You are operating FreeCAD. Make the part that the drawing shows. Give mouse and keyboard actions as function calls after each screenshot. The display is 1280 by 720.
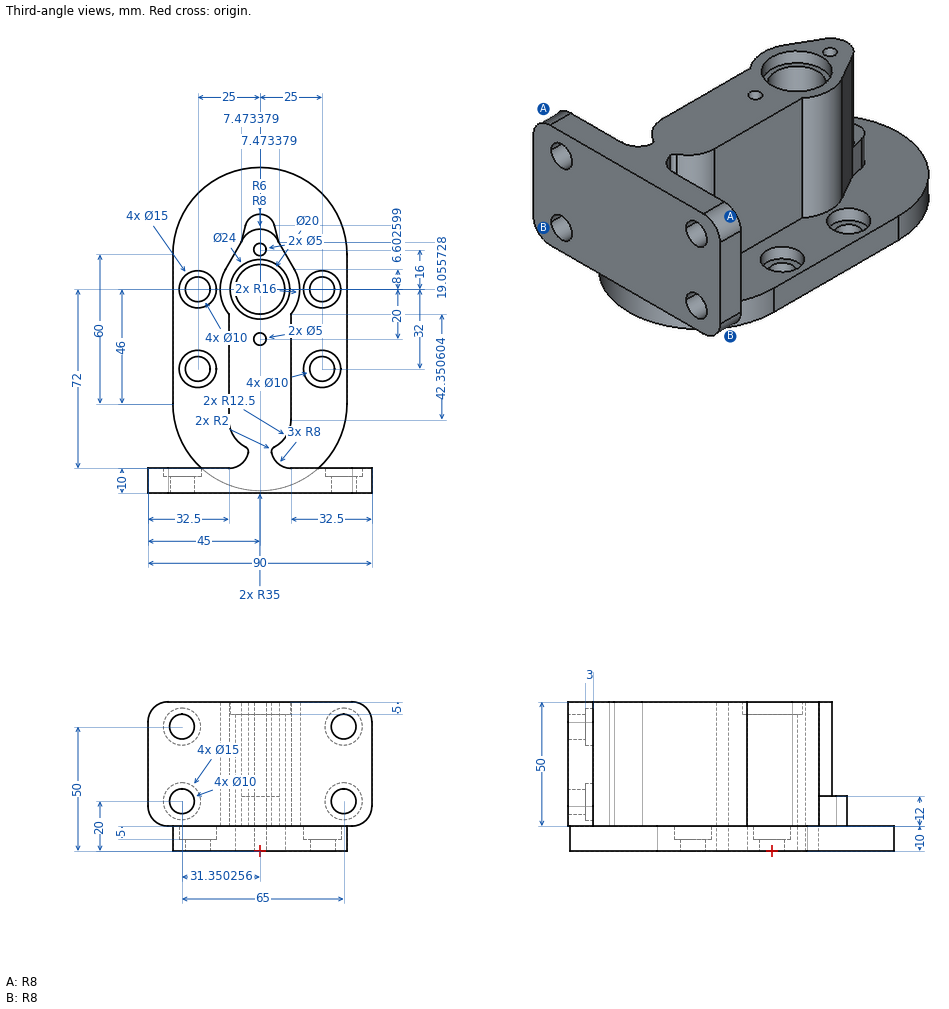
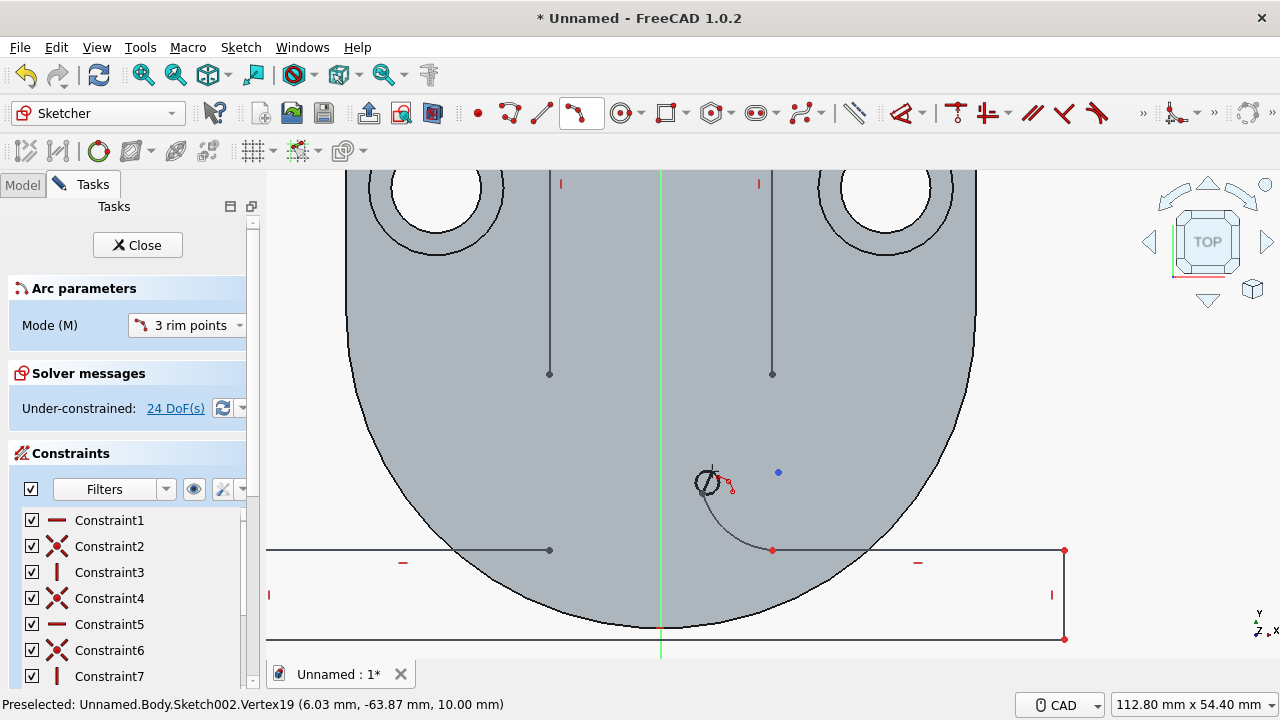
scroll(704, 479, up, 8)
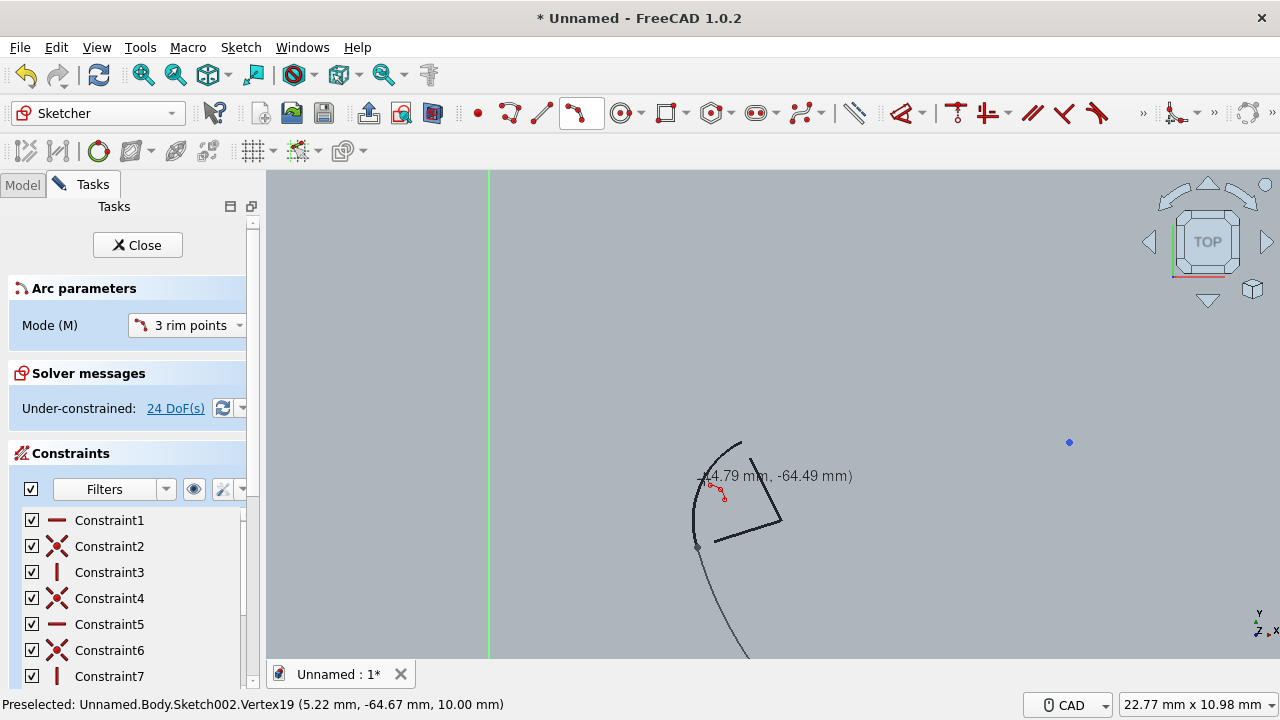
click(704, 476)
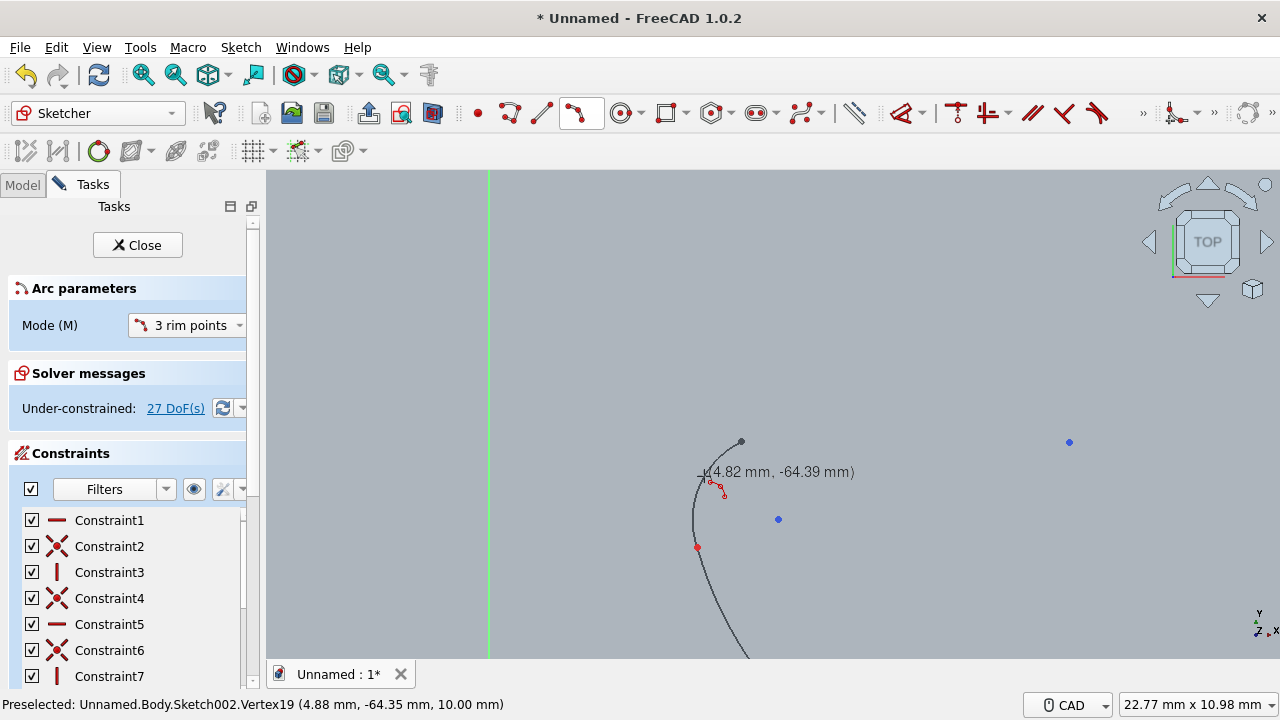
scroll(718, 513, down, 14)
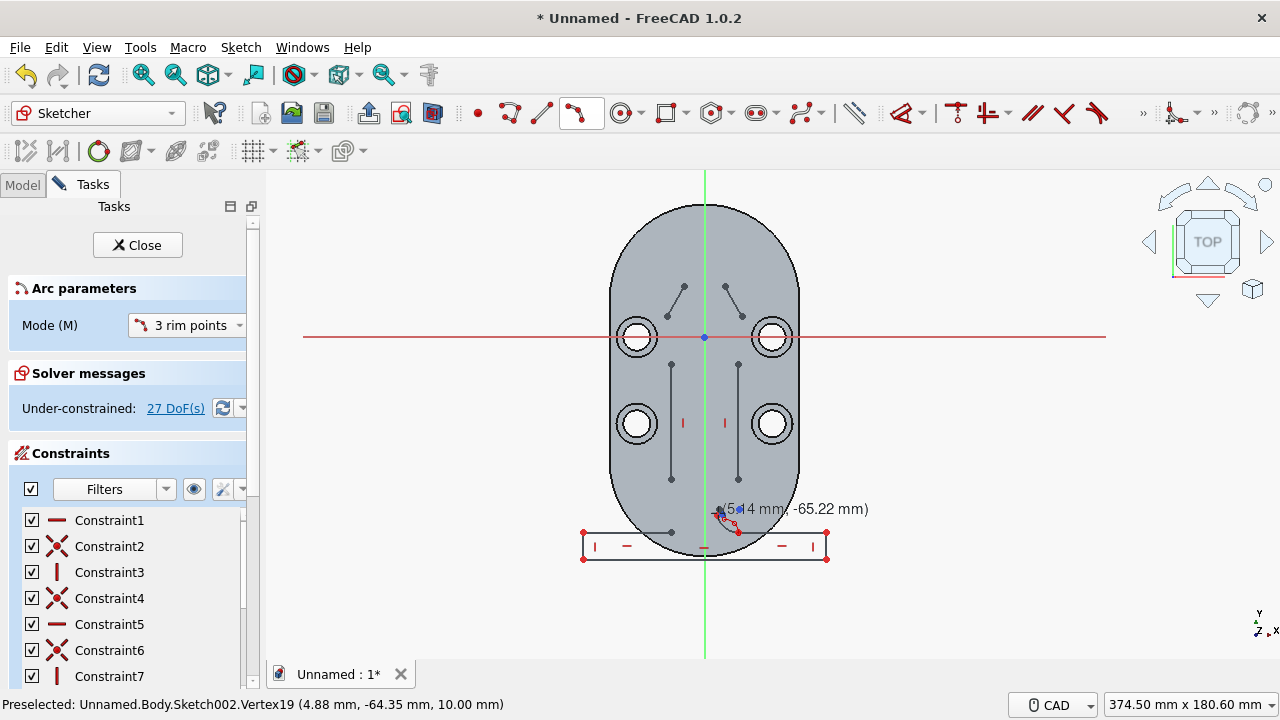
scroll(720, 509, up, 6)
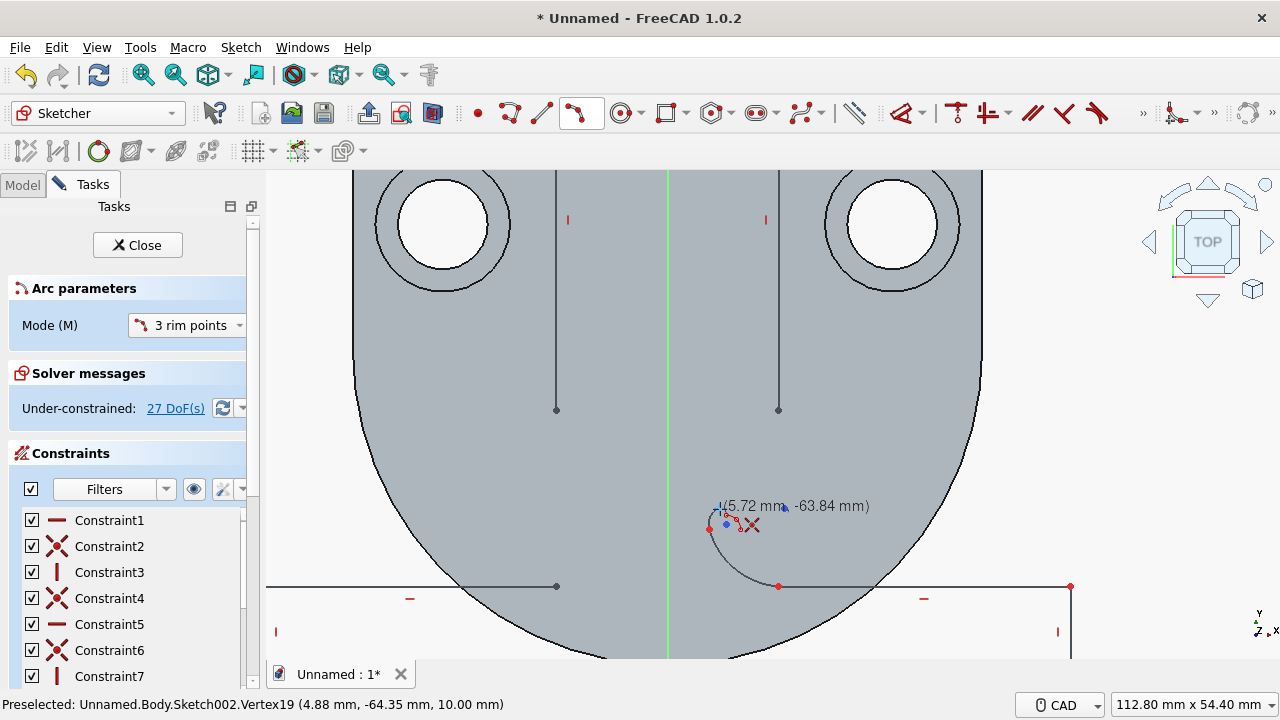
click(719, 508)
click(779, 411)
click(763, 466)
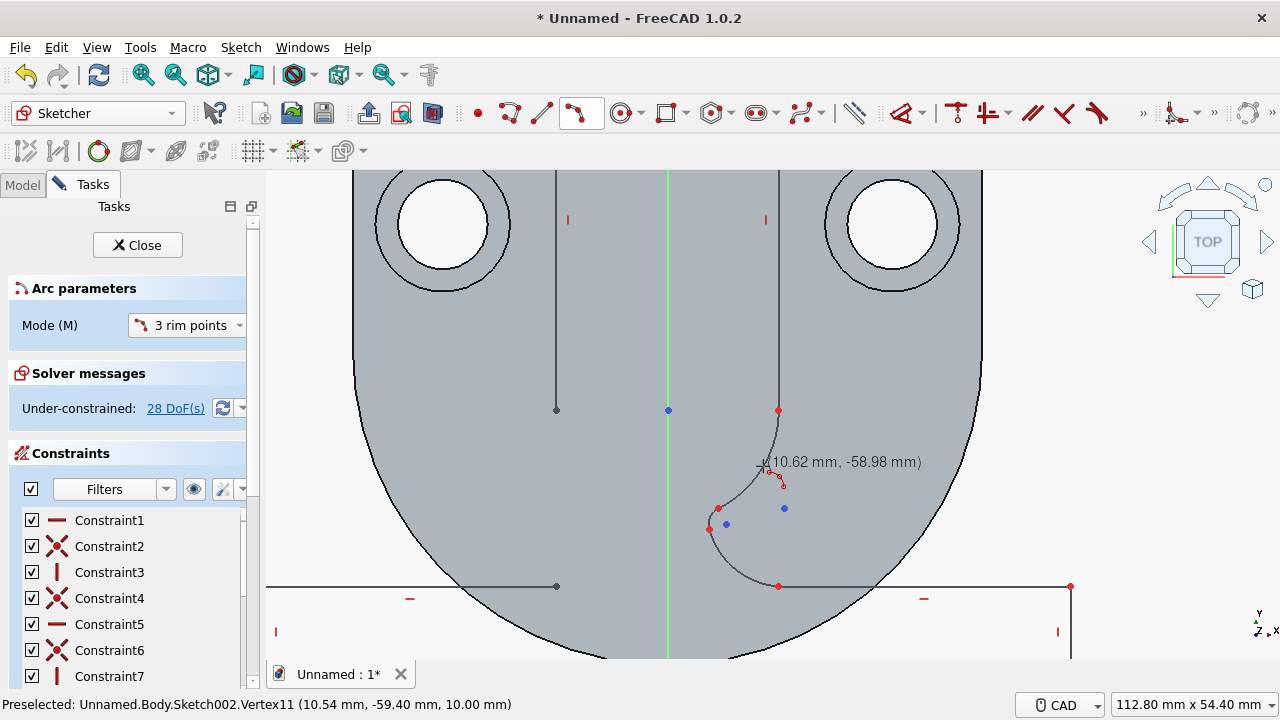
scroll(720, 508, down, 6)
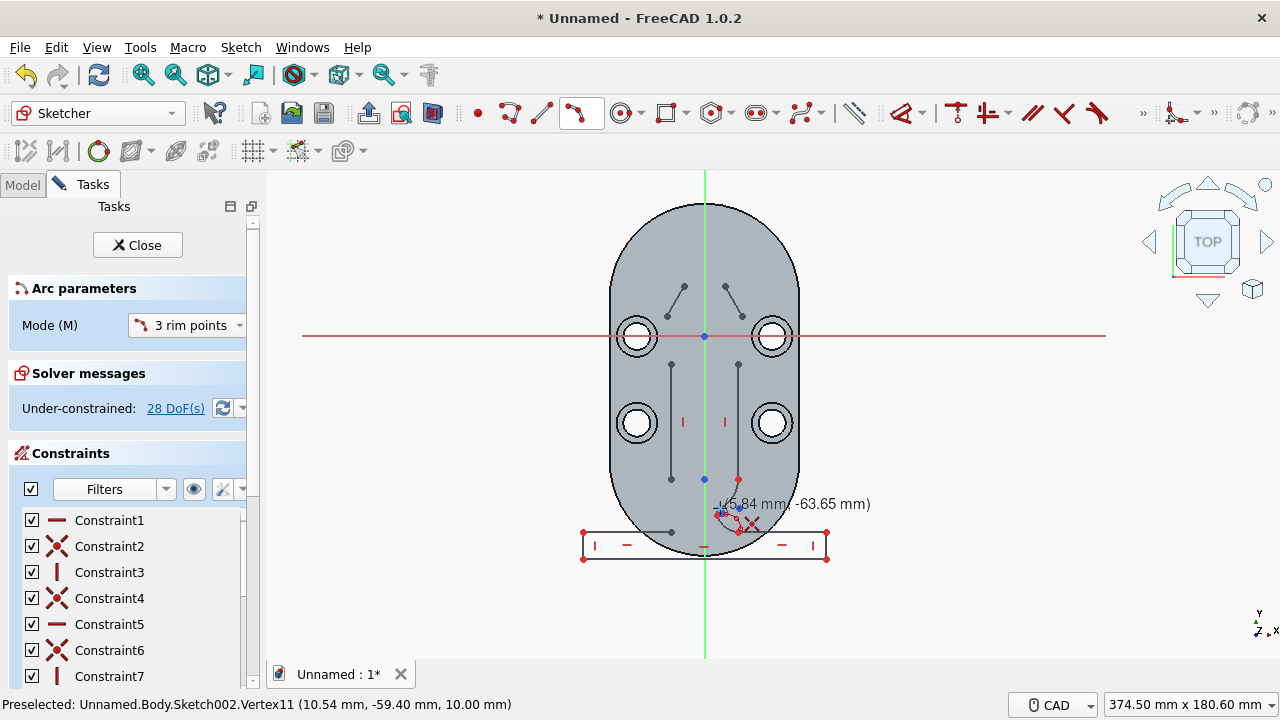
click(738, 364)
click(742, 316)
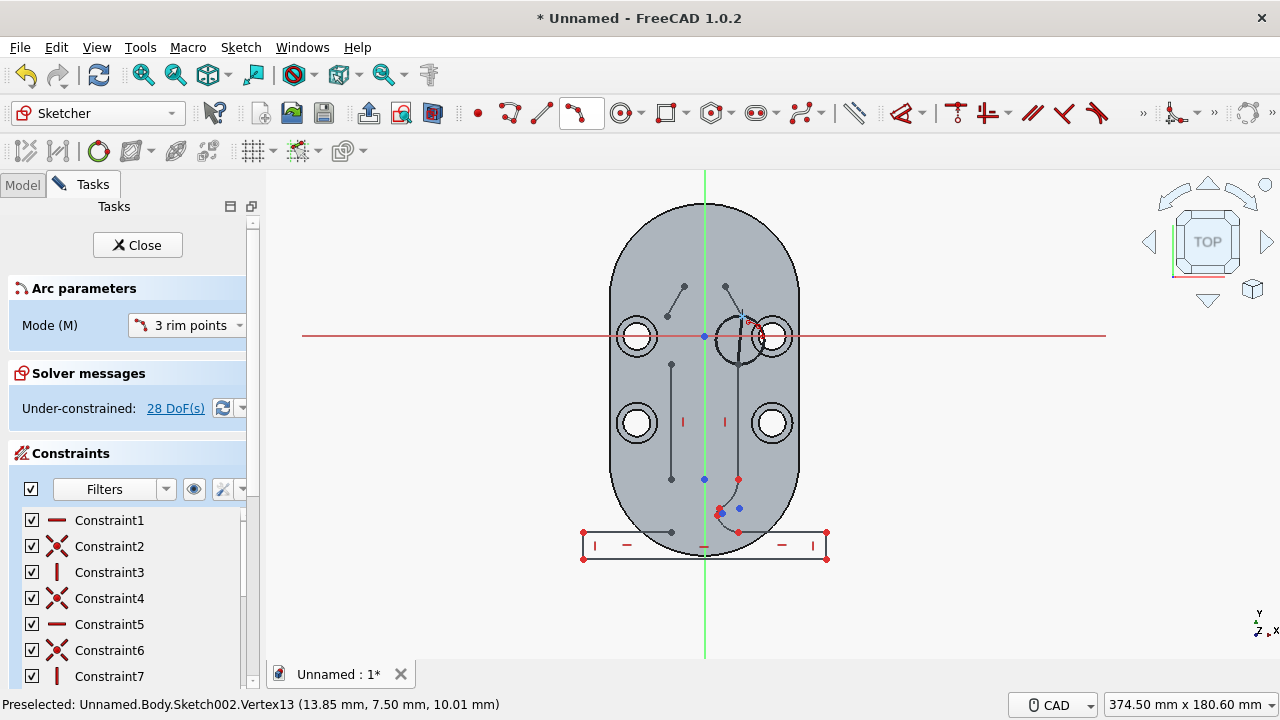
scroll(747, 345, up, 4)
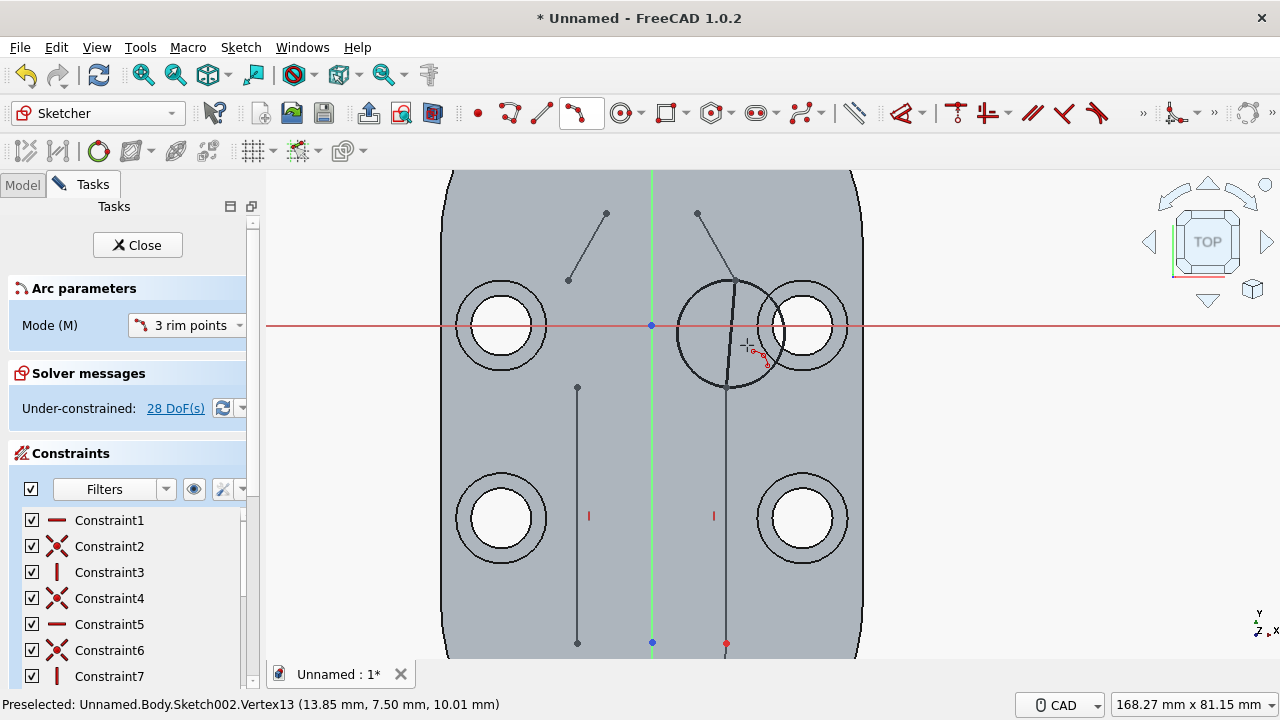
click(746, 344)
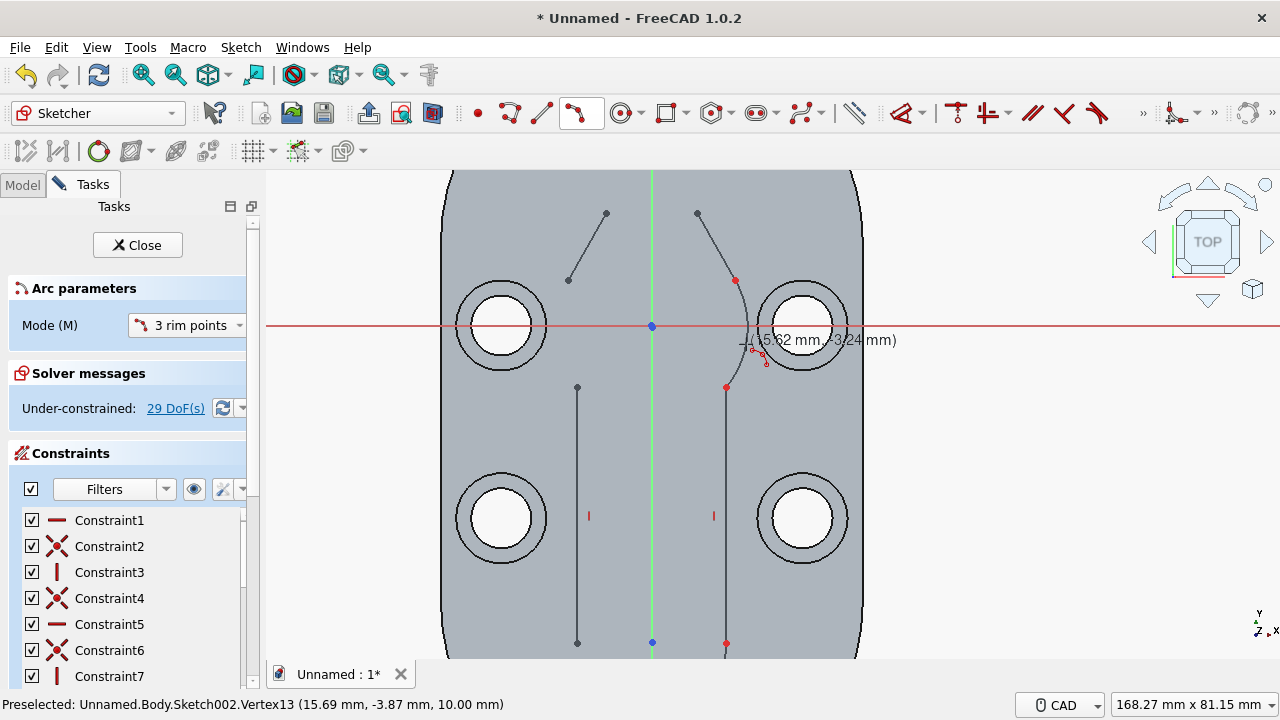
click(697, 214)
click(606, 214)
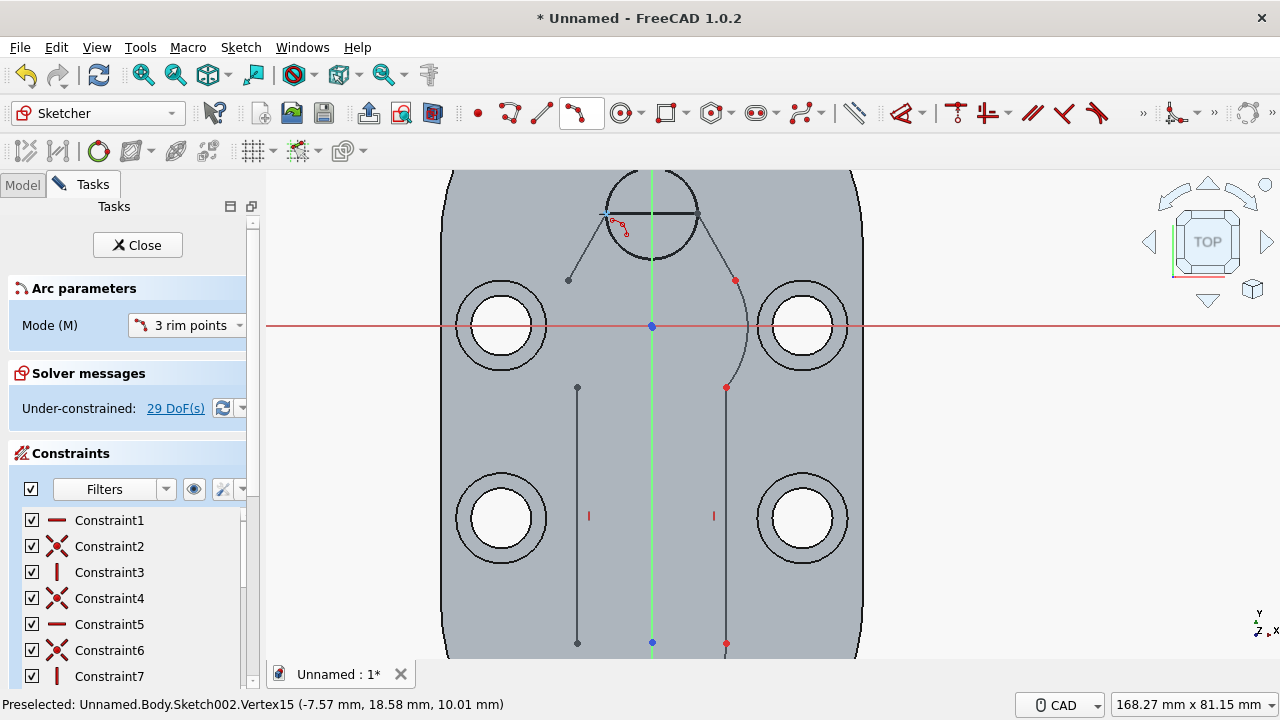
scroll(747, 345, down, 4)